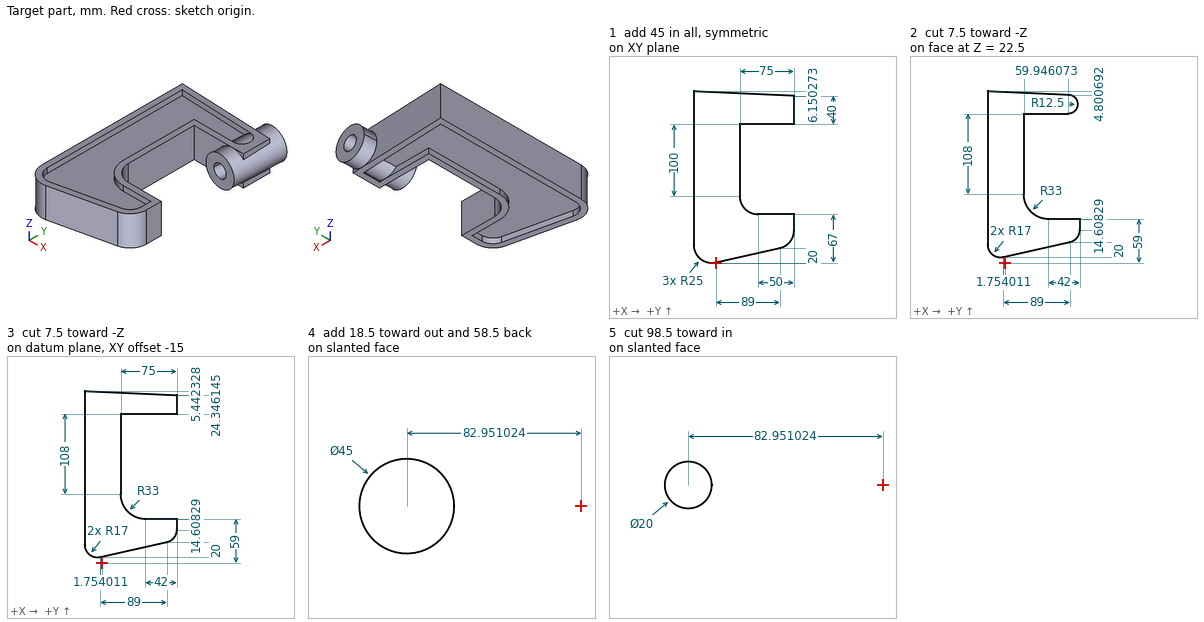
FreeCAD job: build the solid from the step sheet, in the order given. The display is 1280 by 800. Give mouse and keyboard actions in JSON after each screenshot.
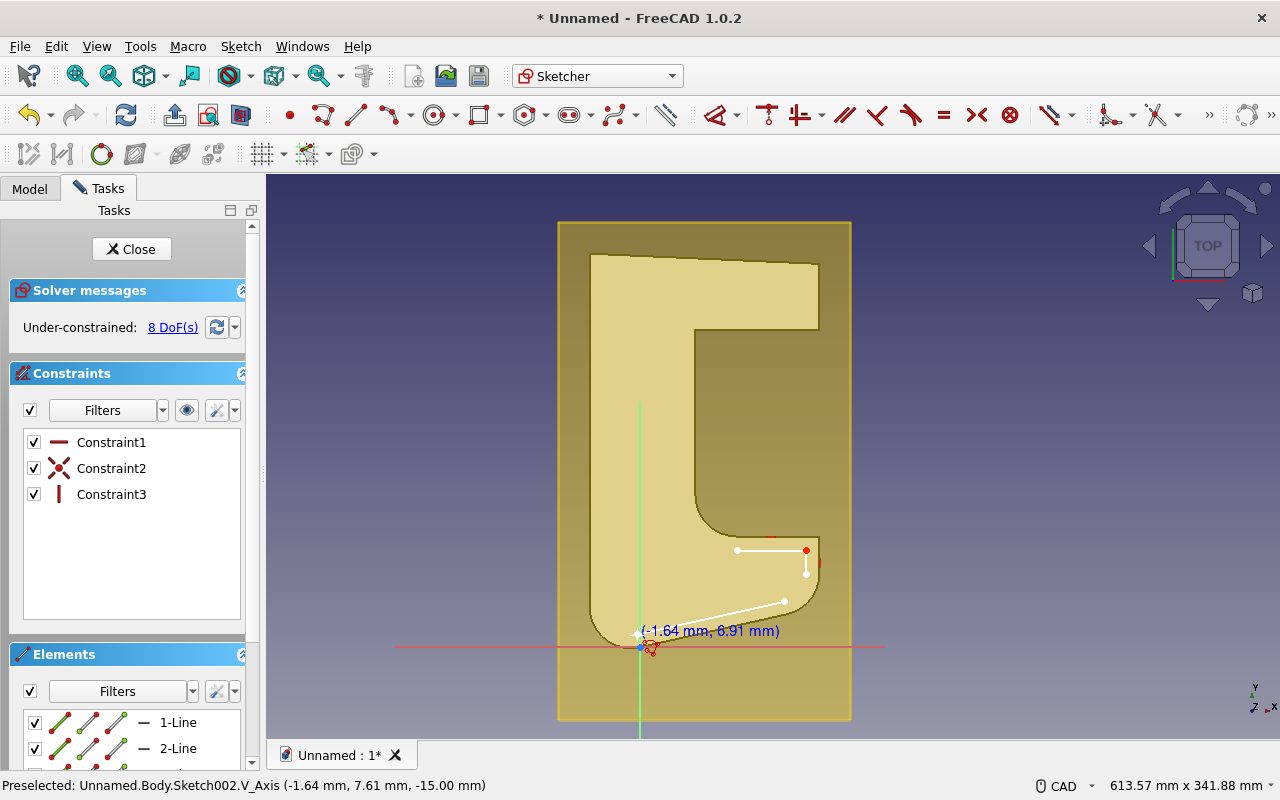
{"action": "left_click", "coordinate": [603, 607]}
{"action": "left_click", "coordinate": [603, 268]}
{"action": "left_click", "coordinate": [806, 279]}
{"action": "left_click", "coordinate": [806, 317]}
{"action": "left_click", "coordinate": [682, 317]}
{"action": "left_click", "coordinate": [682, 495]}
{"action": "right_click", "coordinate": [682, 495]}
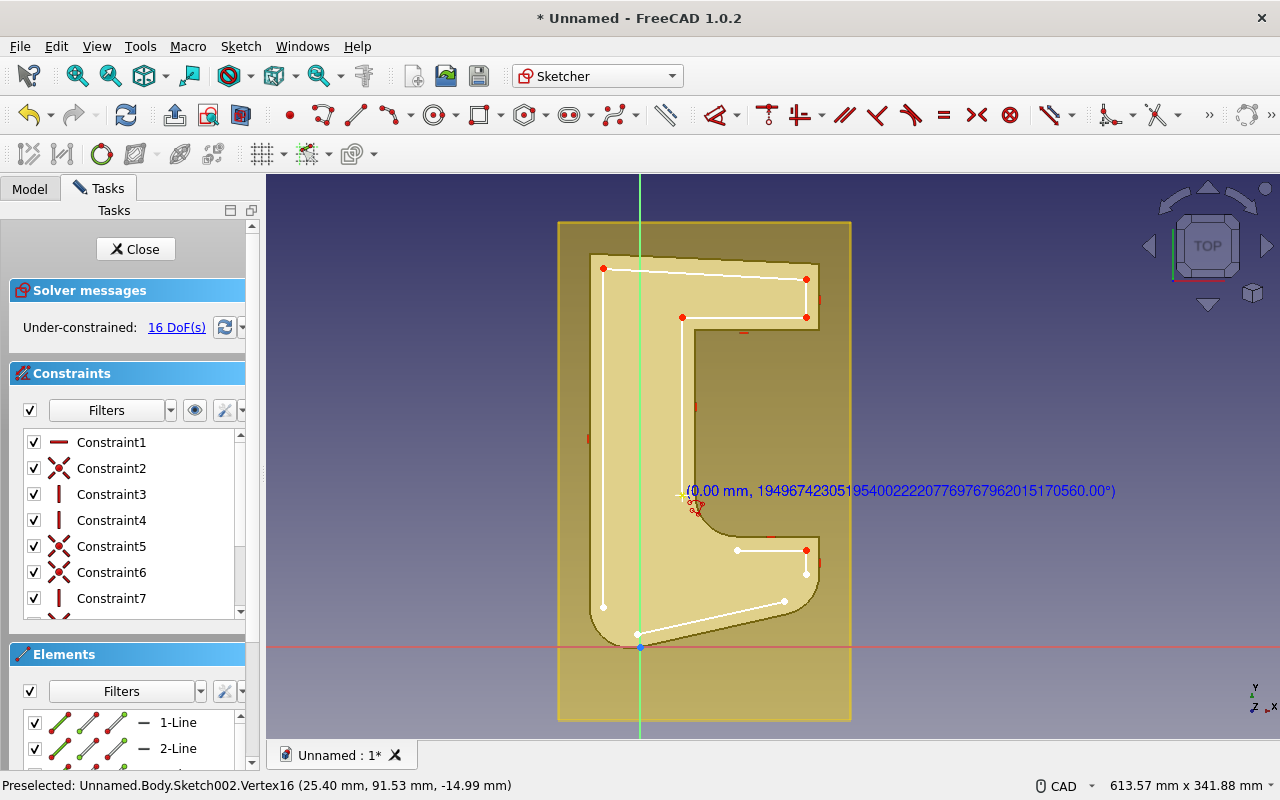
{"action": "left_click", "coordinate": [388, 116]}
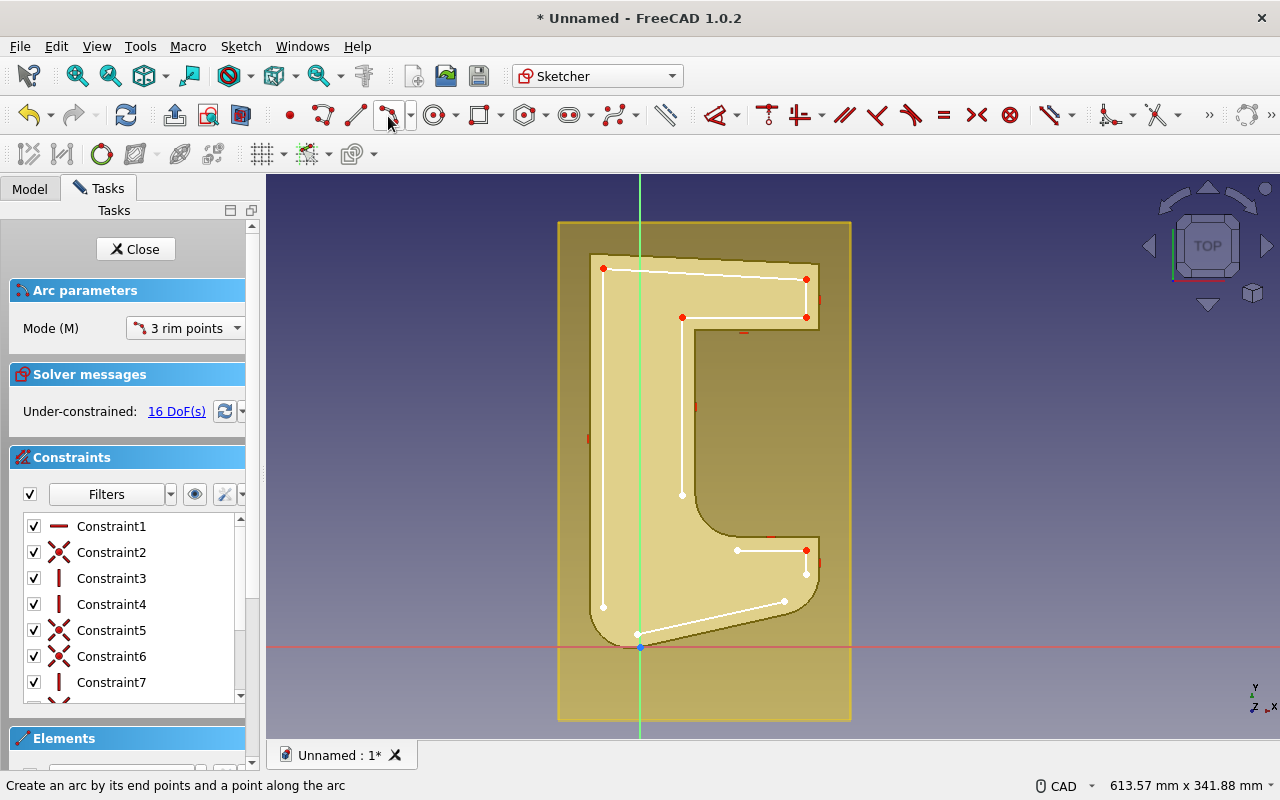
{"action": "scroll", "coordinate": [806, 574], "scroll_direction": "up", "scroll_amount": 2}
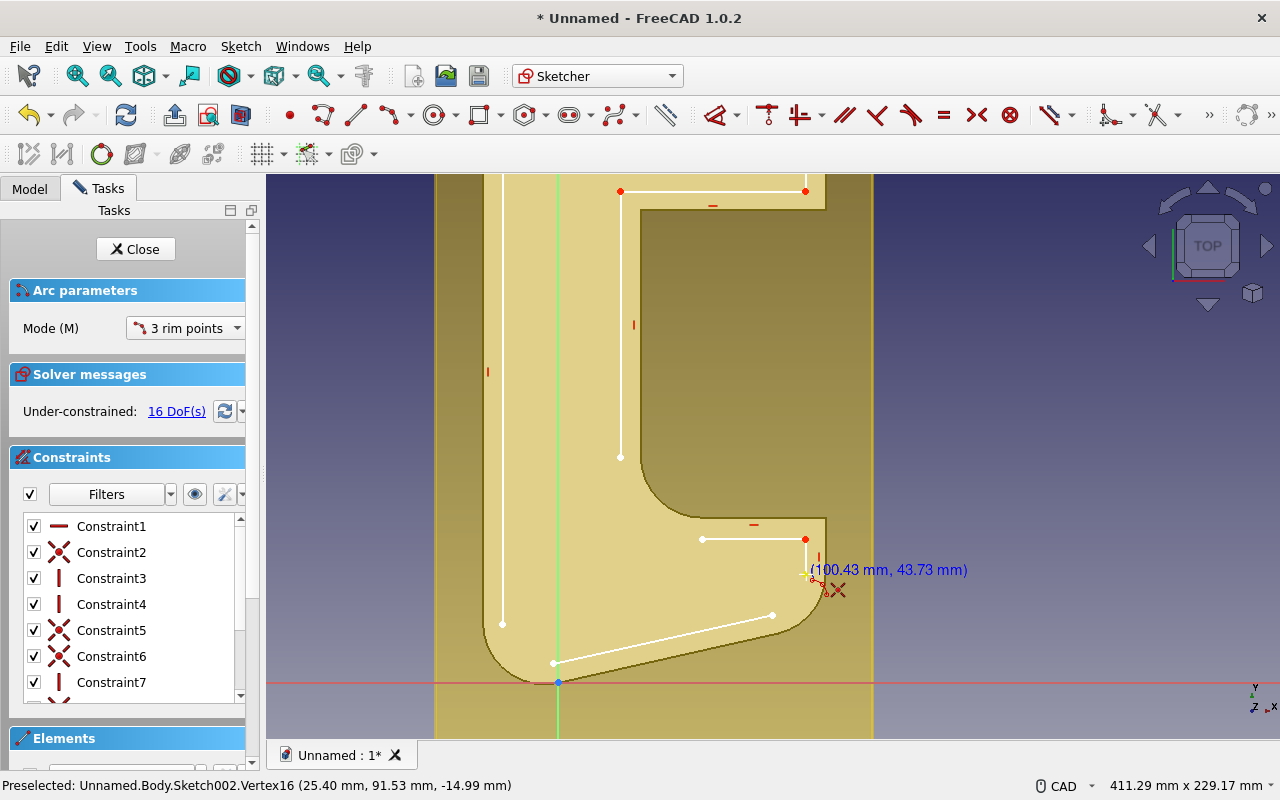
{"action": "left_click", "coordinate": [806, 575]}
{"action": "left_click", "coordinate": [773, 615]}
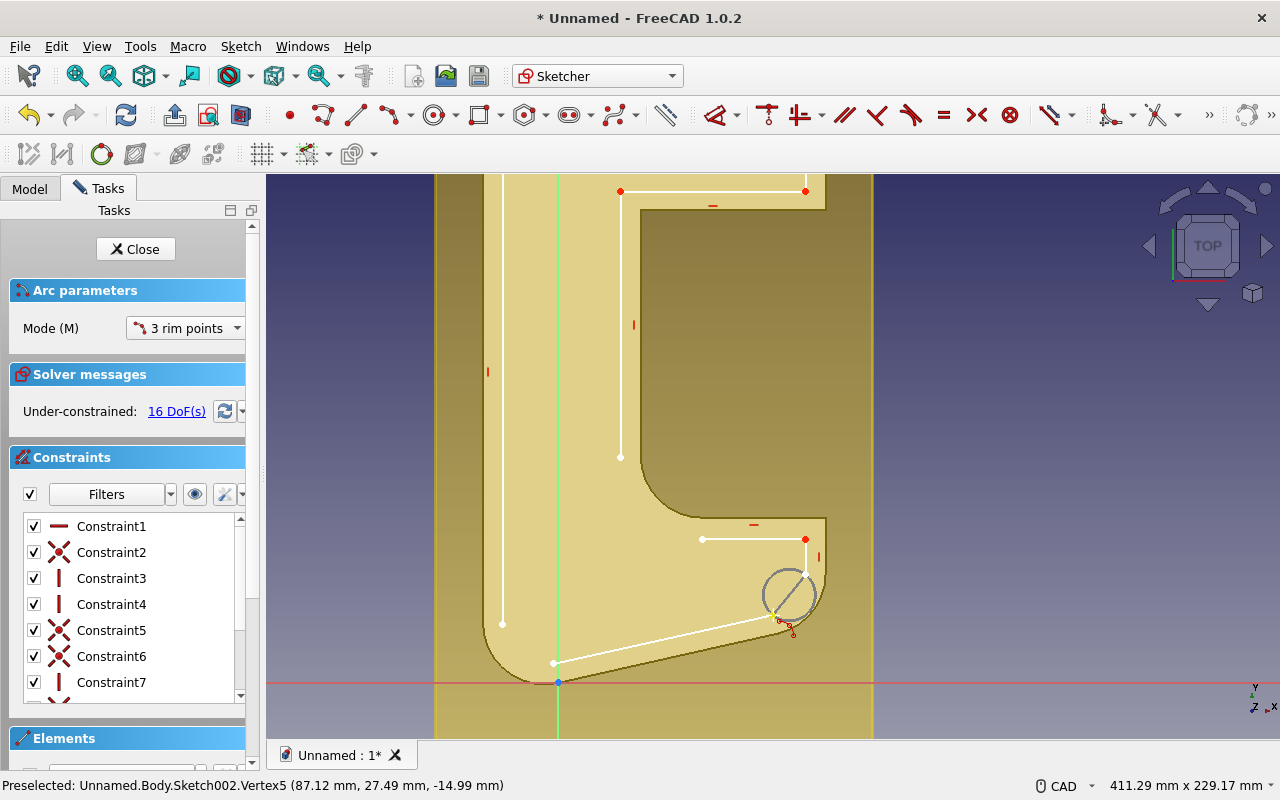
{"action": "scroll", "coordinate": [797, 600], "scroll_direction": "up", "scroll_amount": 3}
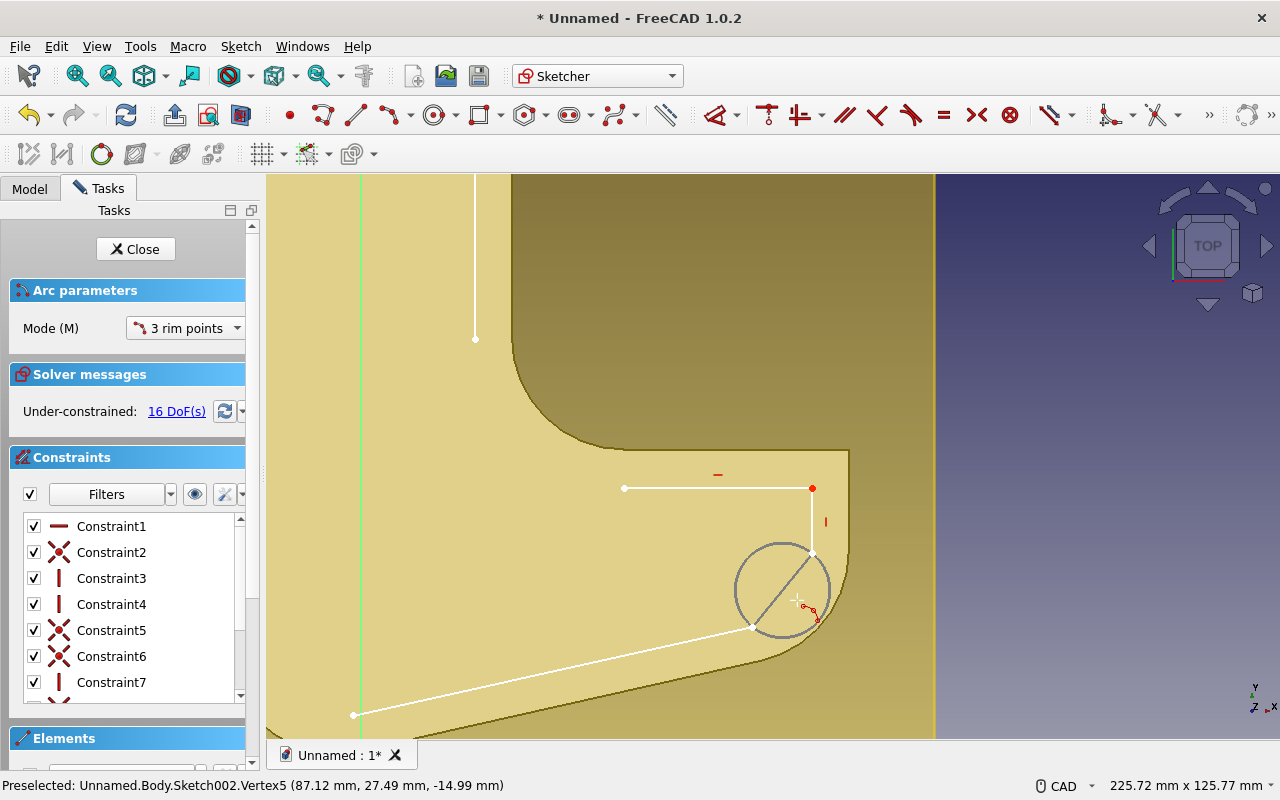
{"action": "left_click", "coordinate": [796, 599]}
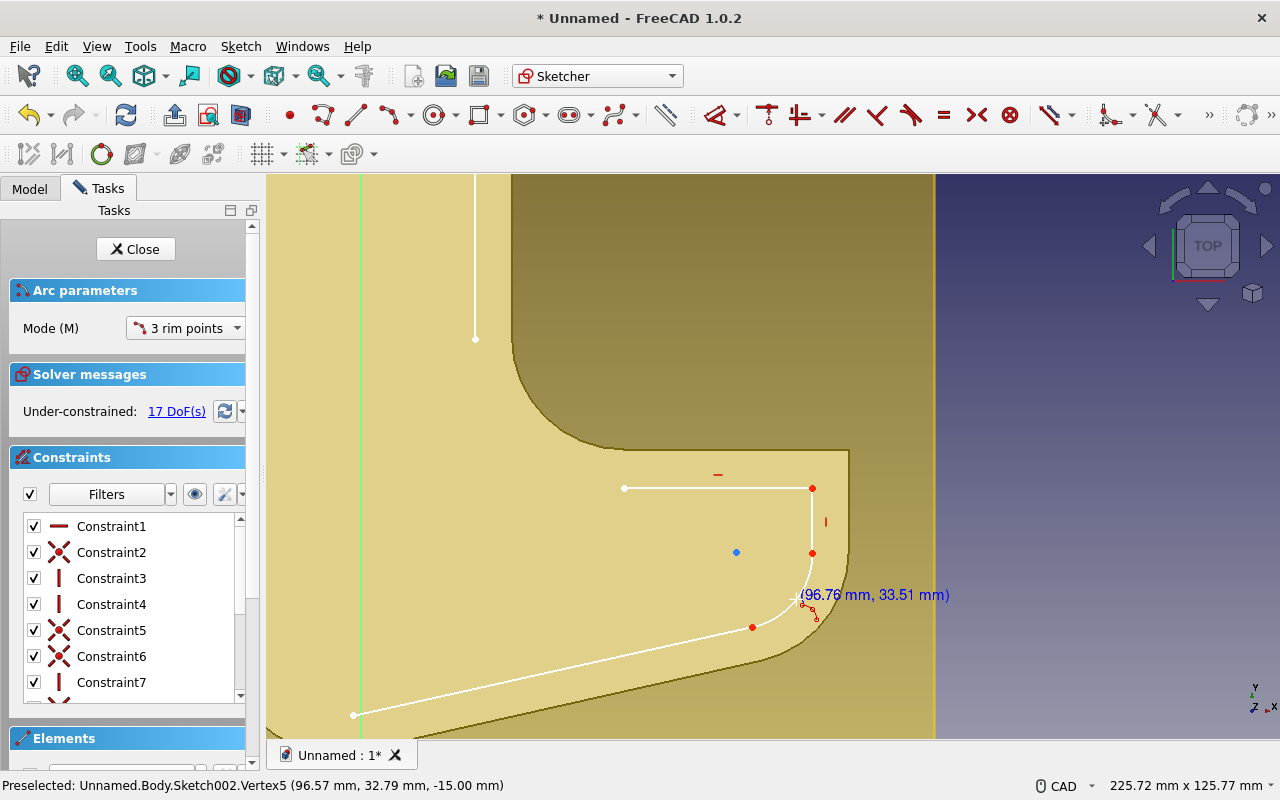
{"action": "scroll", "coordinate": [802, 586], "scroll_direction": "down", "scroll_amount": 5}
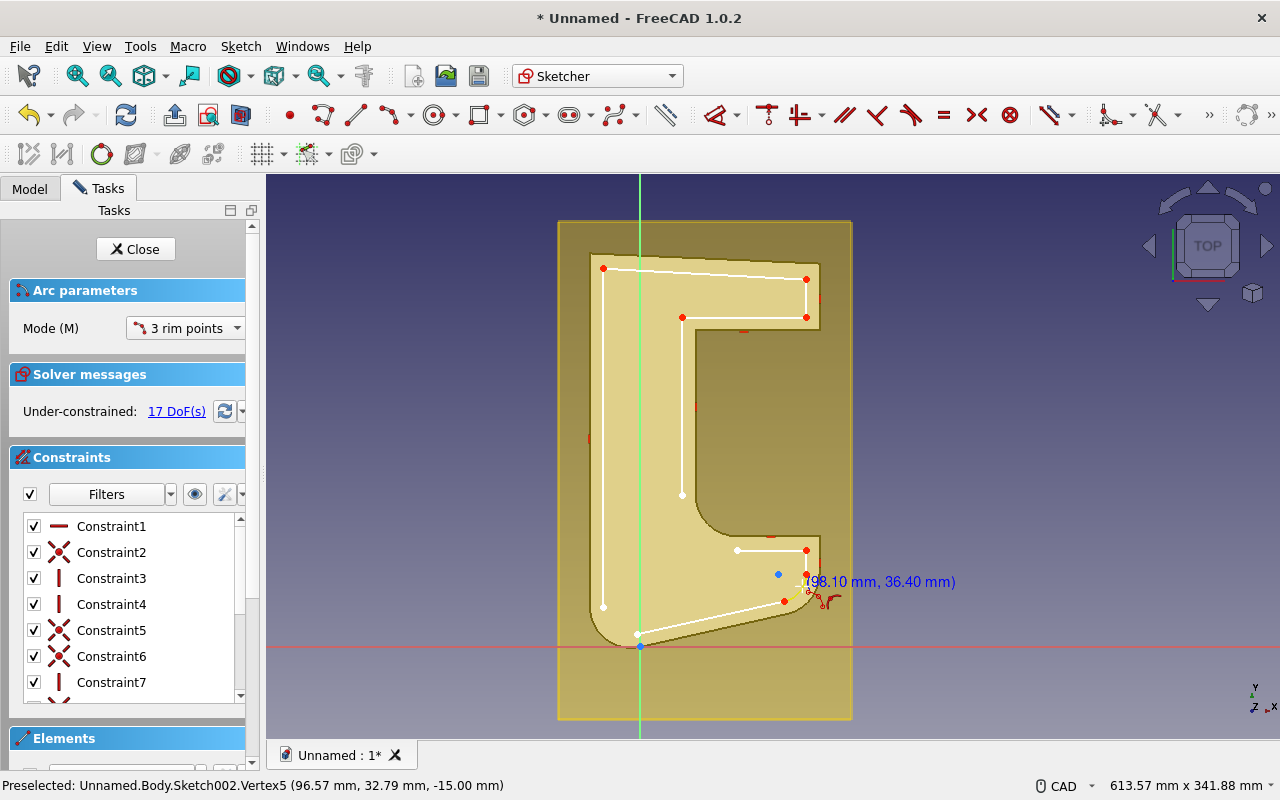
{"action": "scroll", "coordinate": [637, 634], "scroll_direction": "up", "scroll_amount": 9}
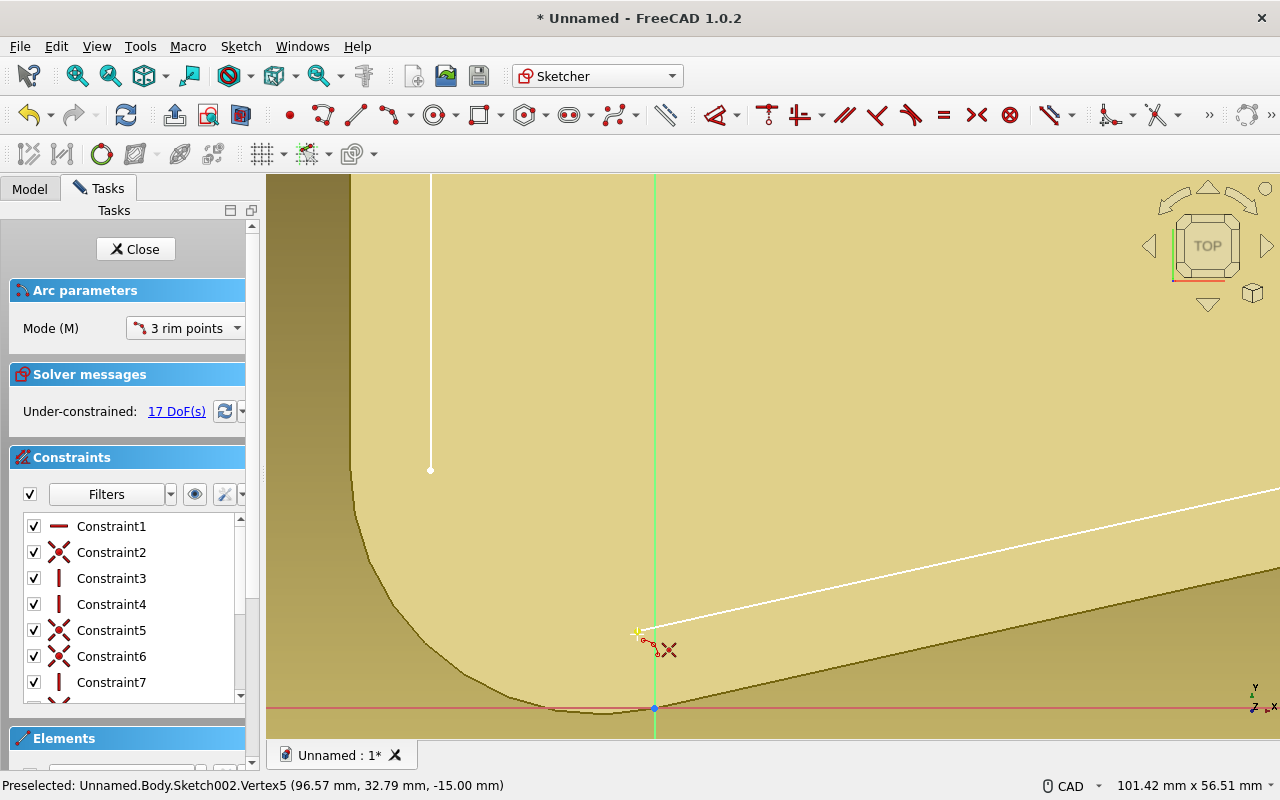
{"action": "left_click", "coordinate": [637, 631]}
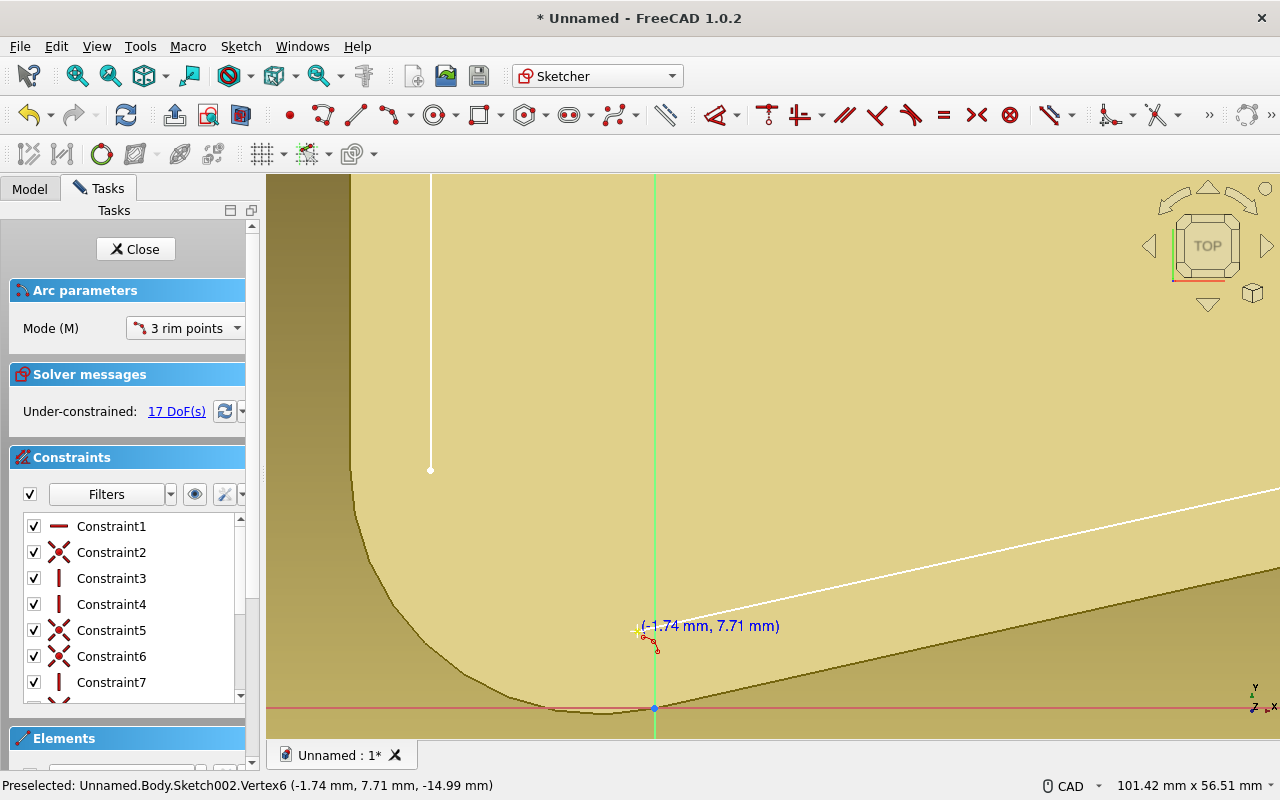
{"action": "scroll", "coordinate": [637, 634], "scroll_direction": "down", "scroll_amount": 9}